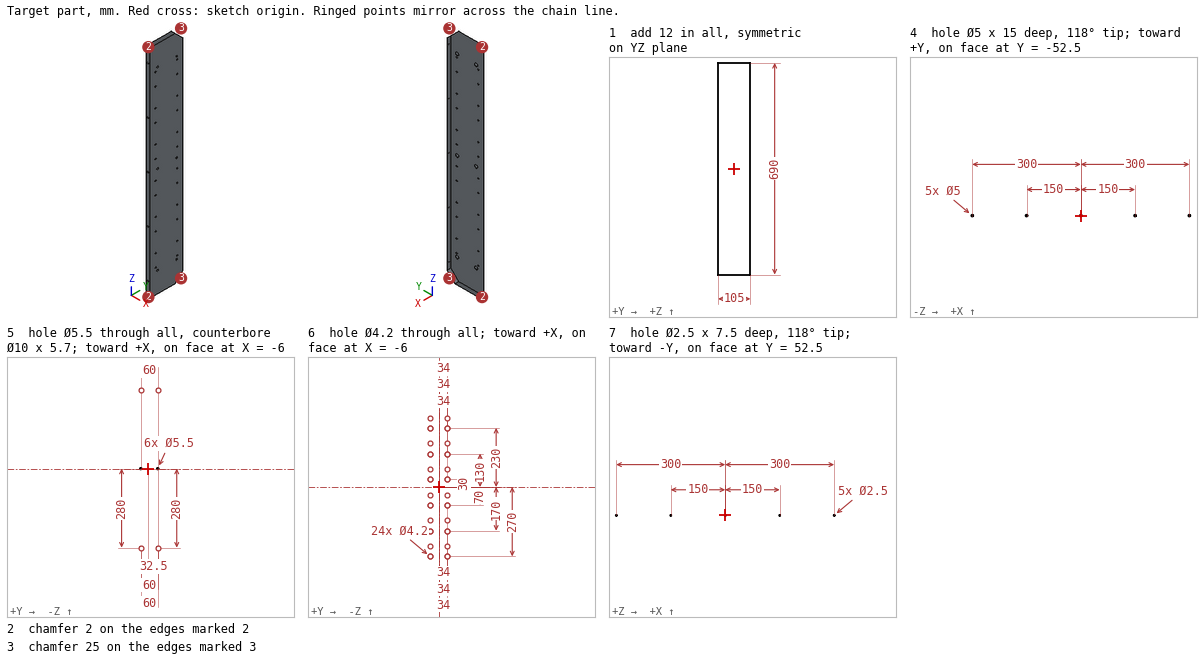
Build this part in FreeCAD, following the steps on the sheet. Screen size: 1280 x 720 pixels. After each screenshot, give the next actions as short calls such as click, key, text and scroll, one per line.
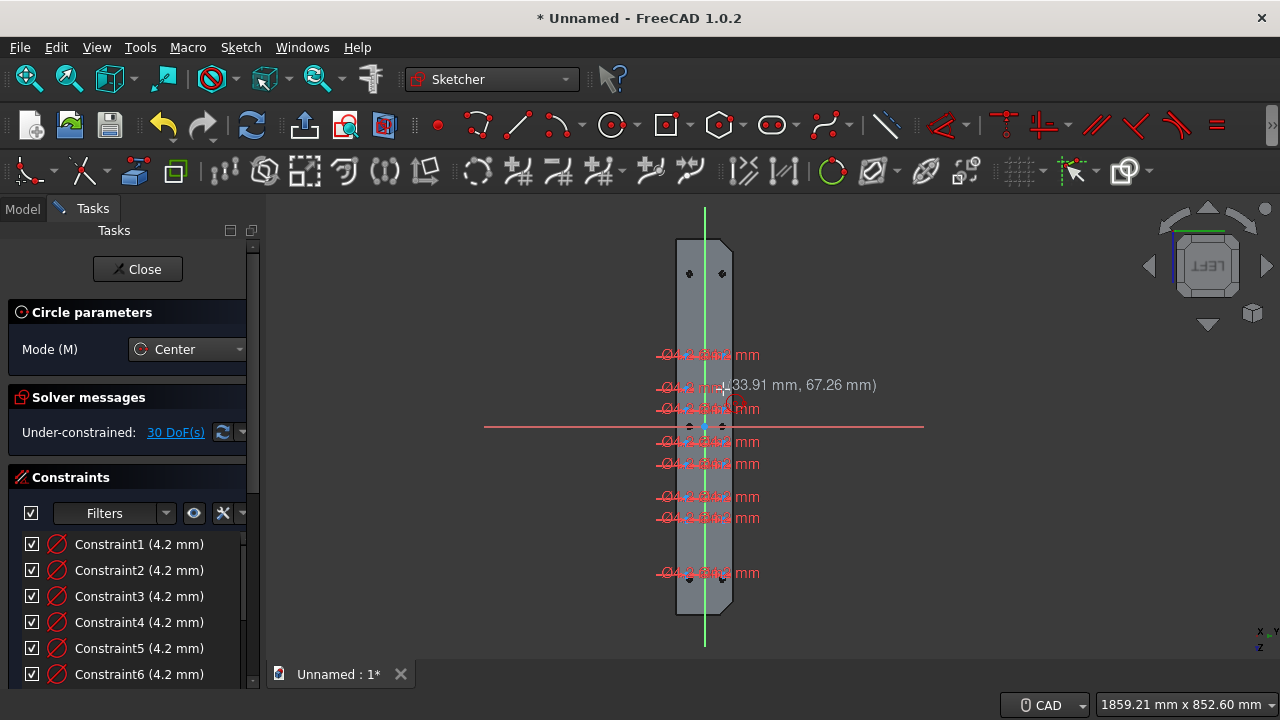
click(723, 389)
move(724, 388)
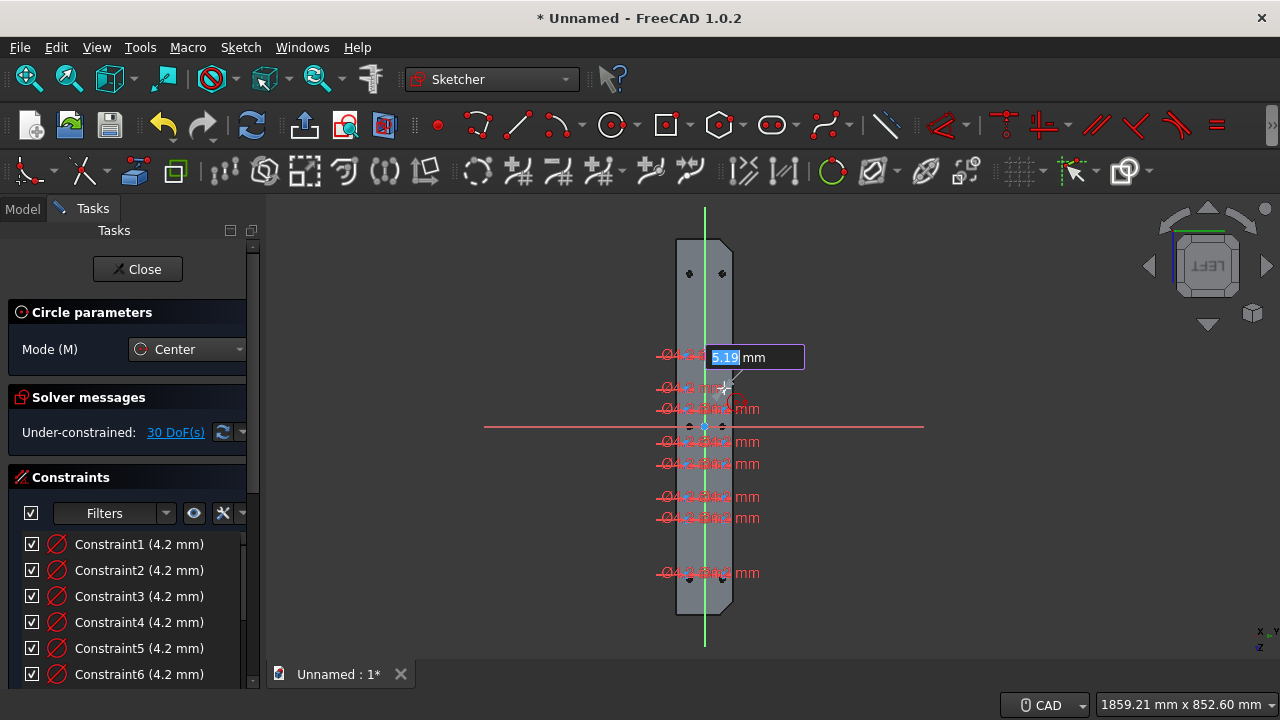
text(4.2)
key(Return)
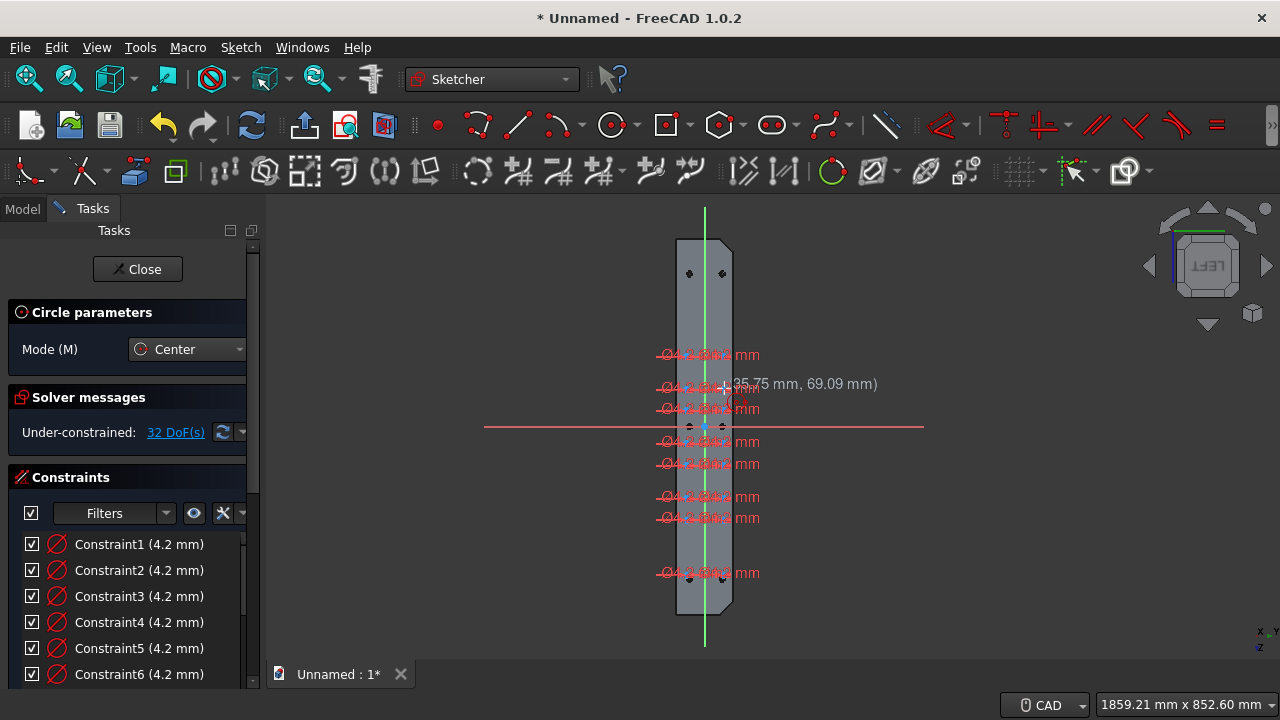
scroll(686, 334, up, 15)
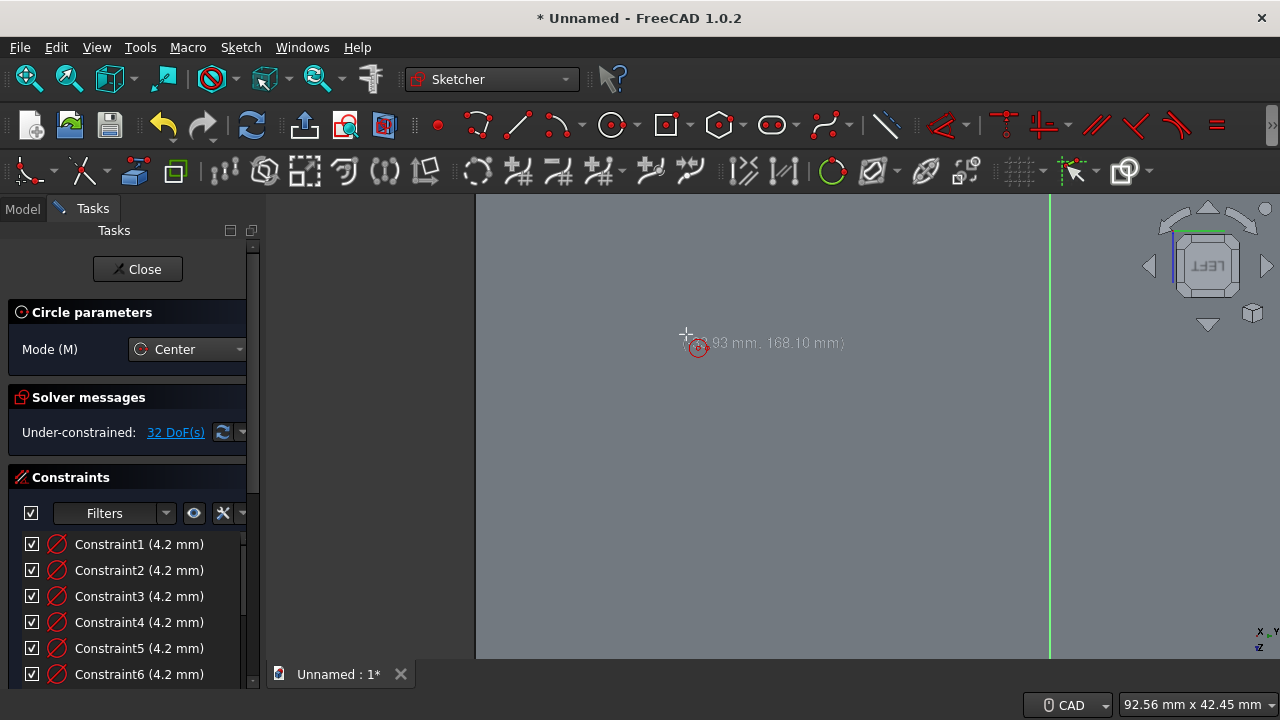
scroll(686, 334, down, 15)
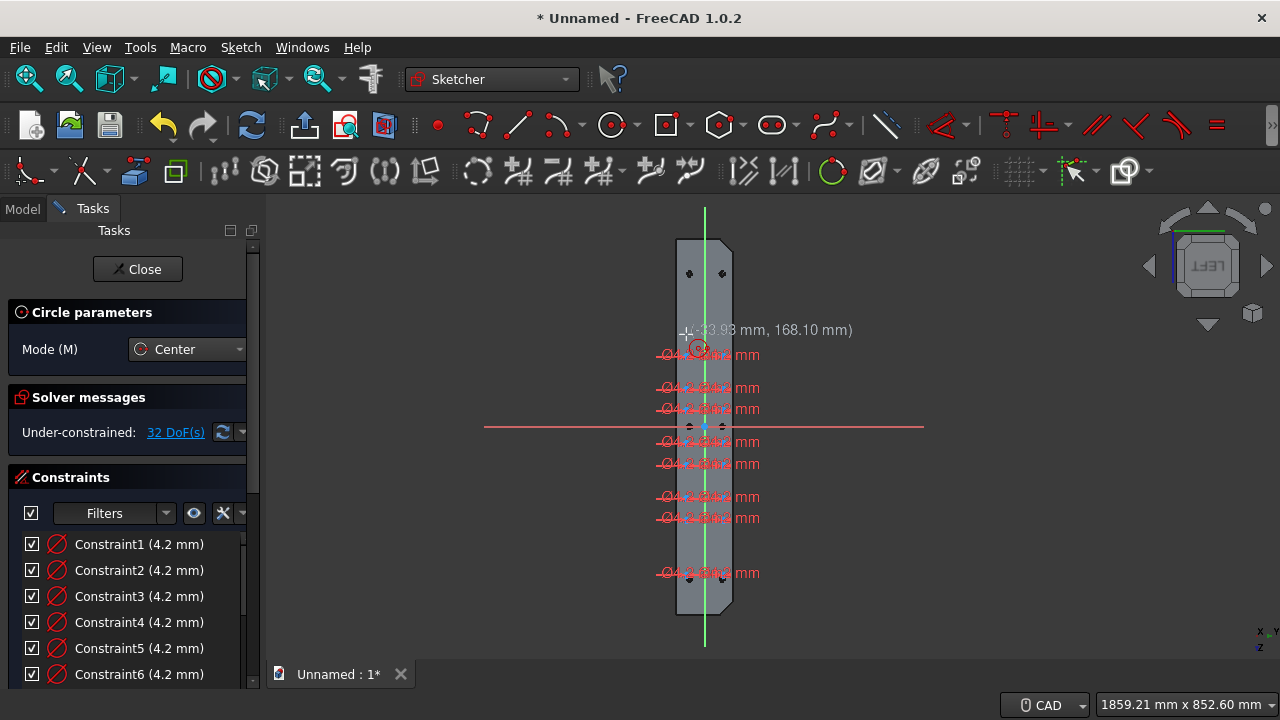
click(686, 334)
move(687, 333)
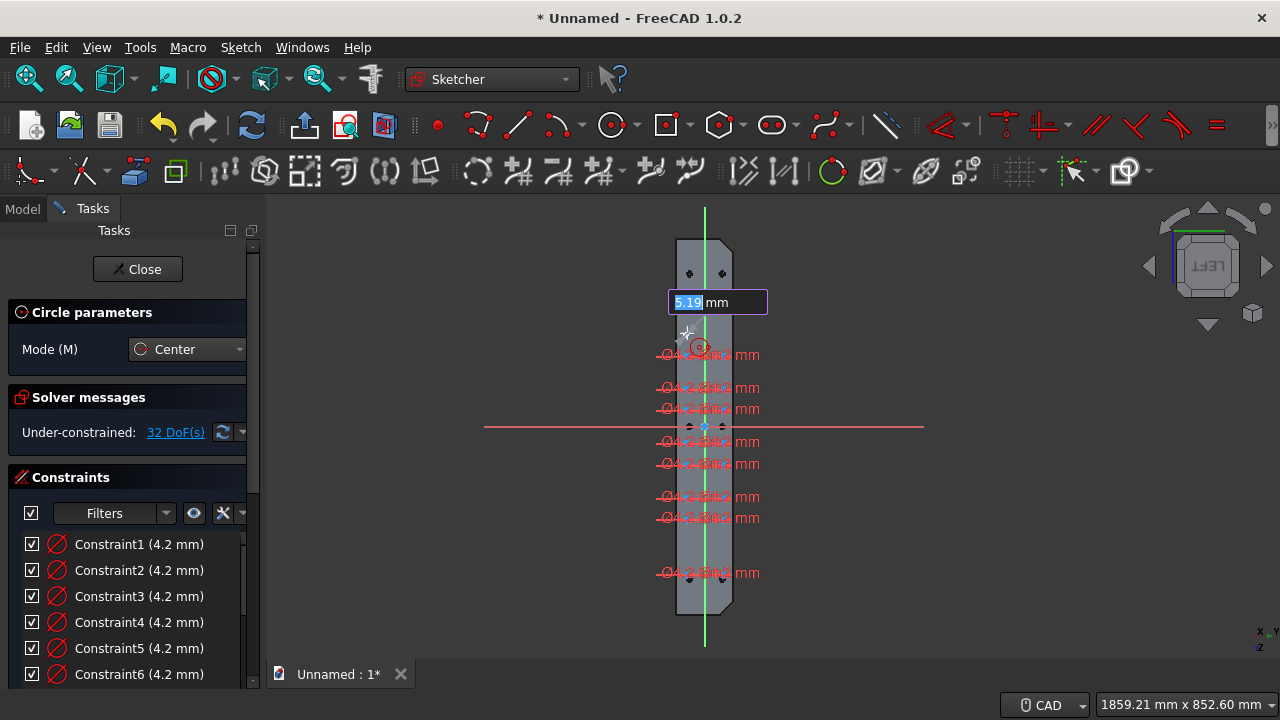
text(4.2)
key(Return)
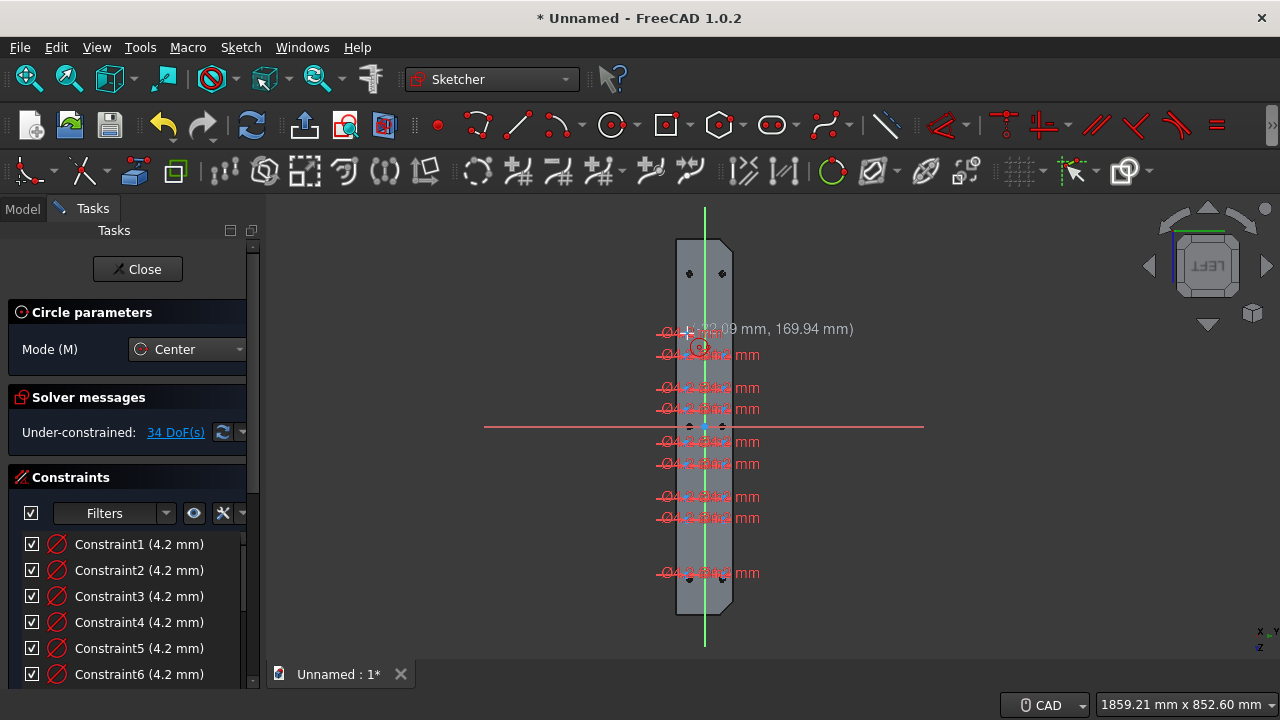
scroll(723, 334, up, 15)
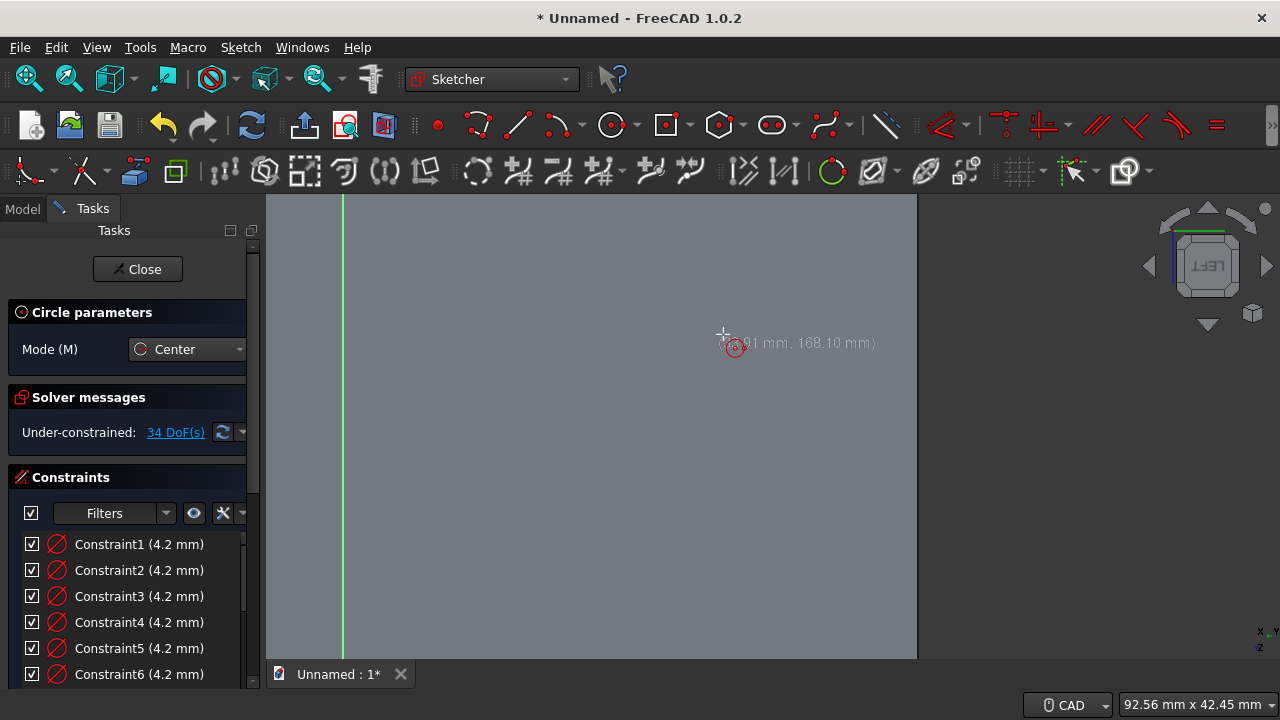
scroll(723, 334, down, 15)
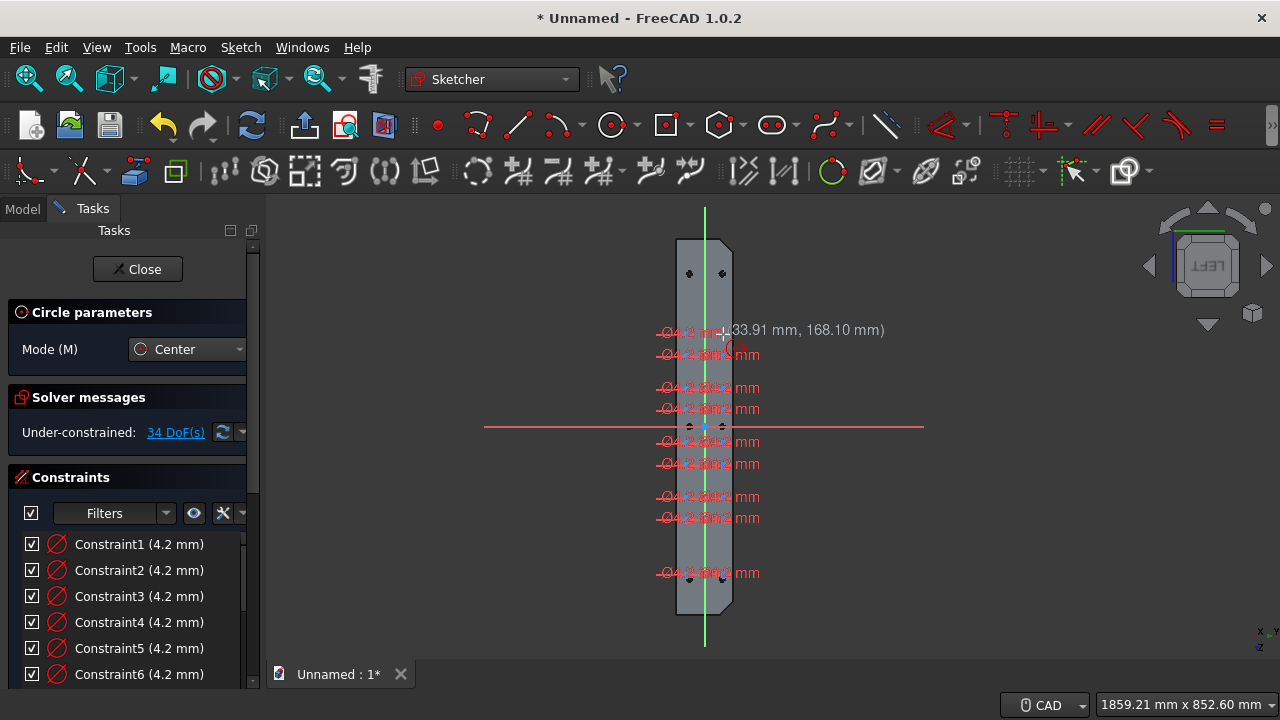
click(723, 334)
move(724, 333)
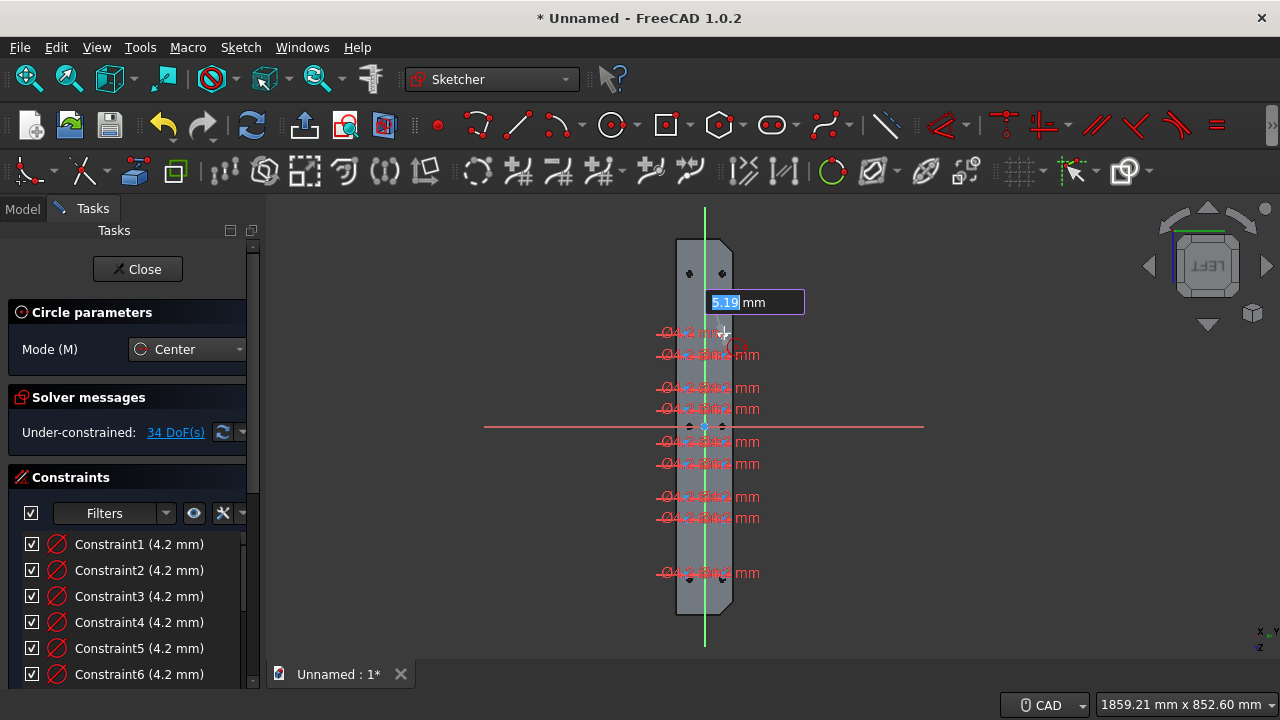
text(4.2)
key(Return)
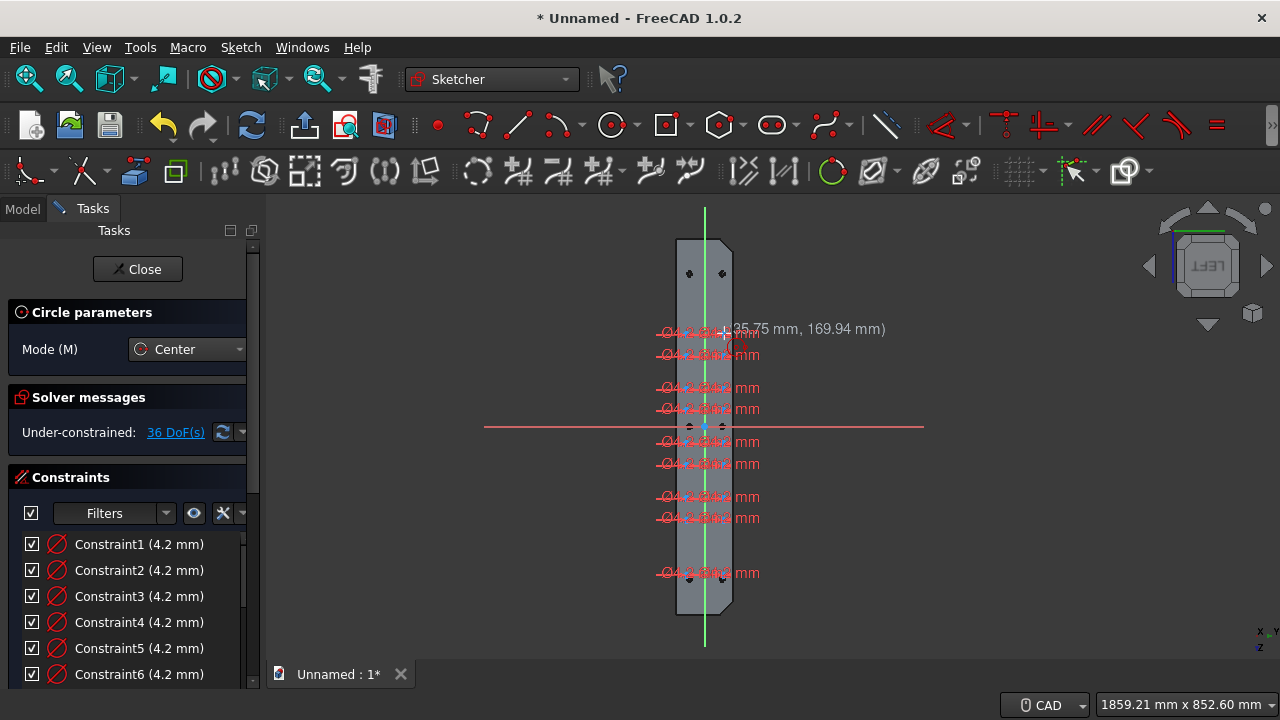
scroll(686, 279, up, 15)